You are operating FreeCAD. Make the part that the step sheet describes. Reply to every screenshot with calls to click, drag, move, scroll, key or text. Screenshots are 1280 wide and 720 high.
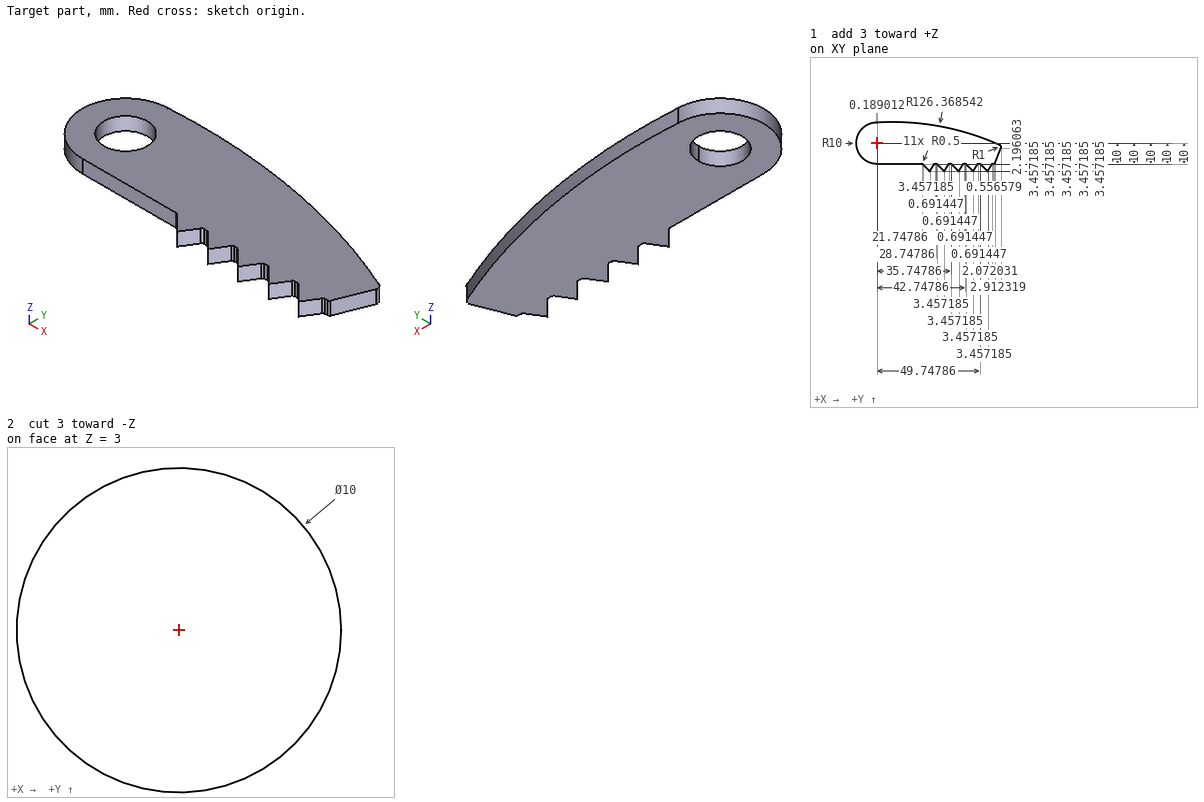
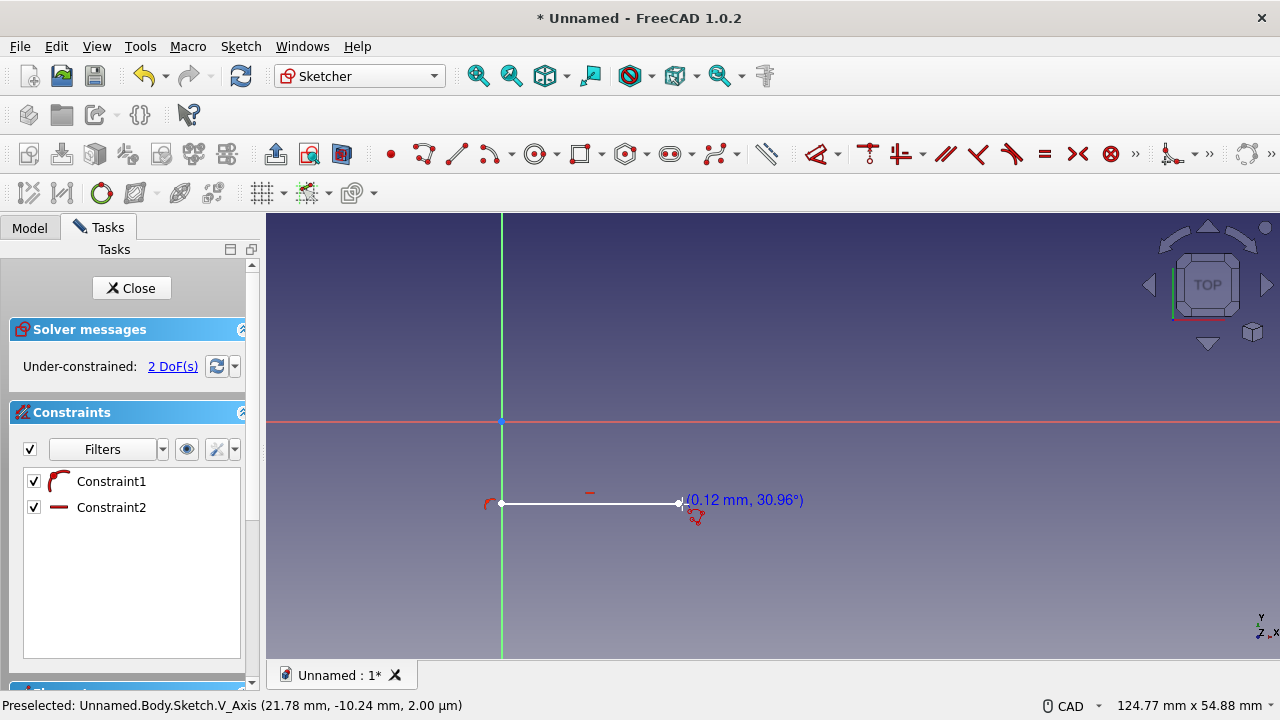
click(710, 532)
click(726, 505)
right_click(726, 505)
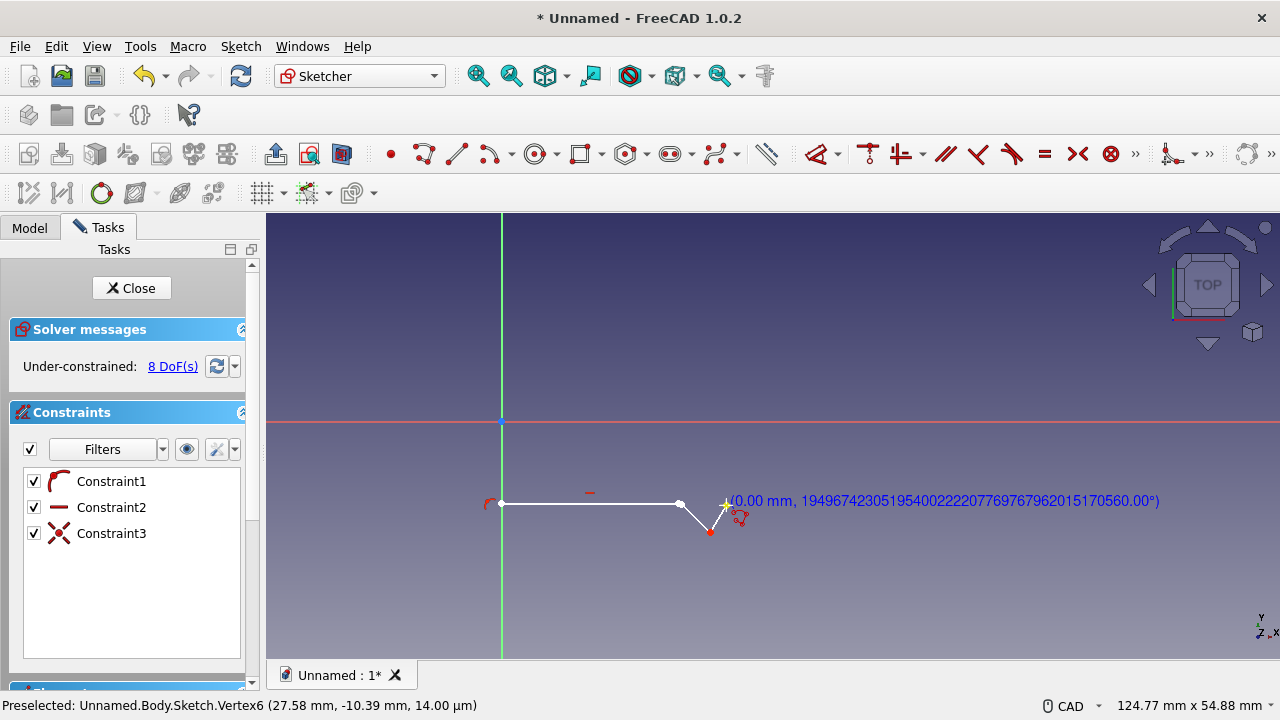
click(457, 154)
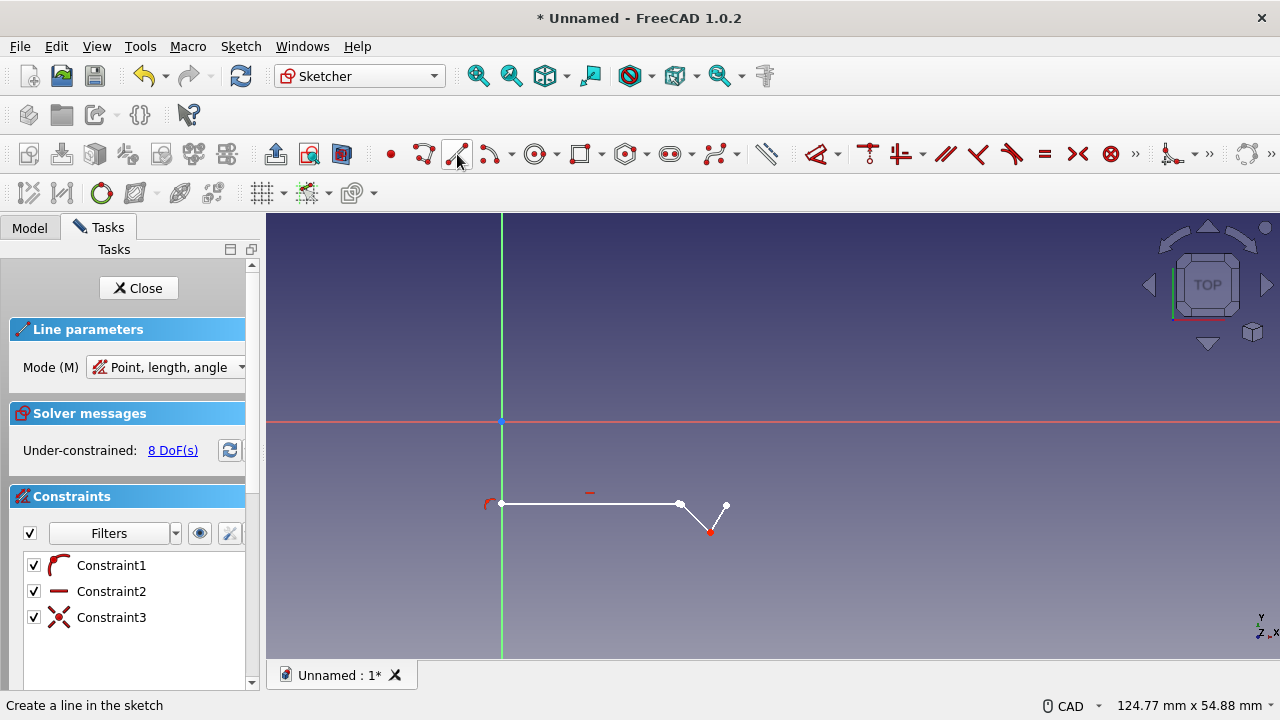
scroll(730, 503, up, 7)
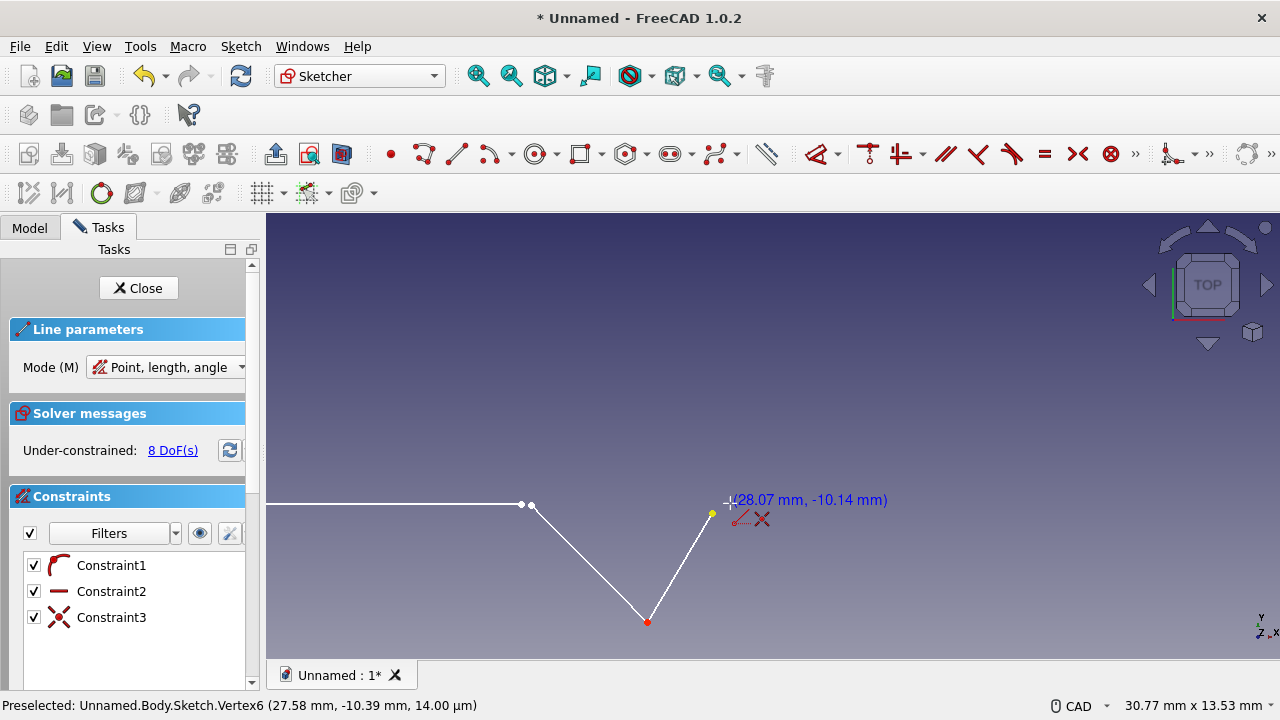
click(728, 500)
click(751, 500)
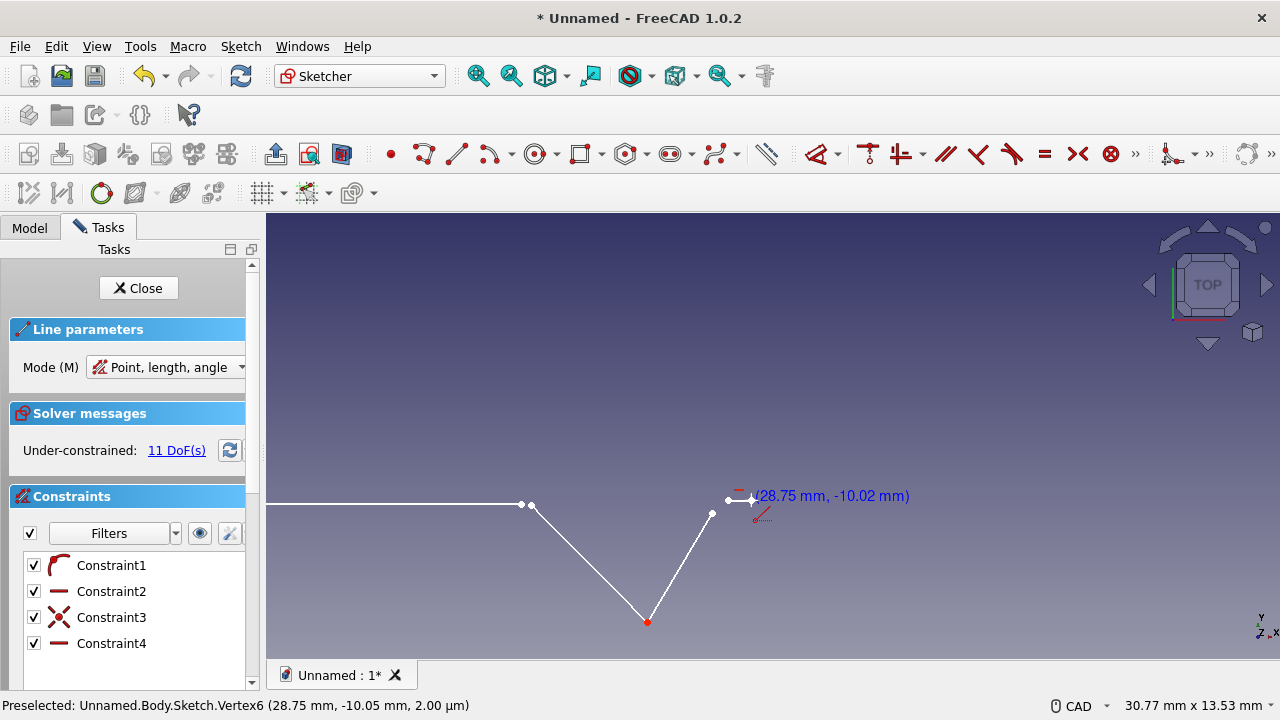
click(424, 154)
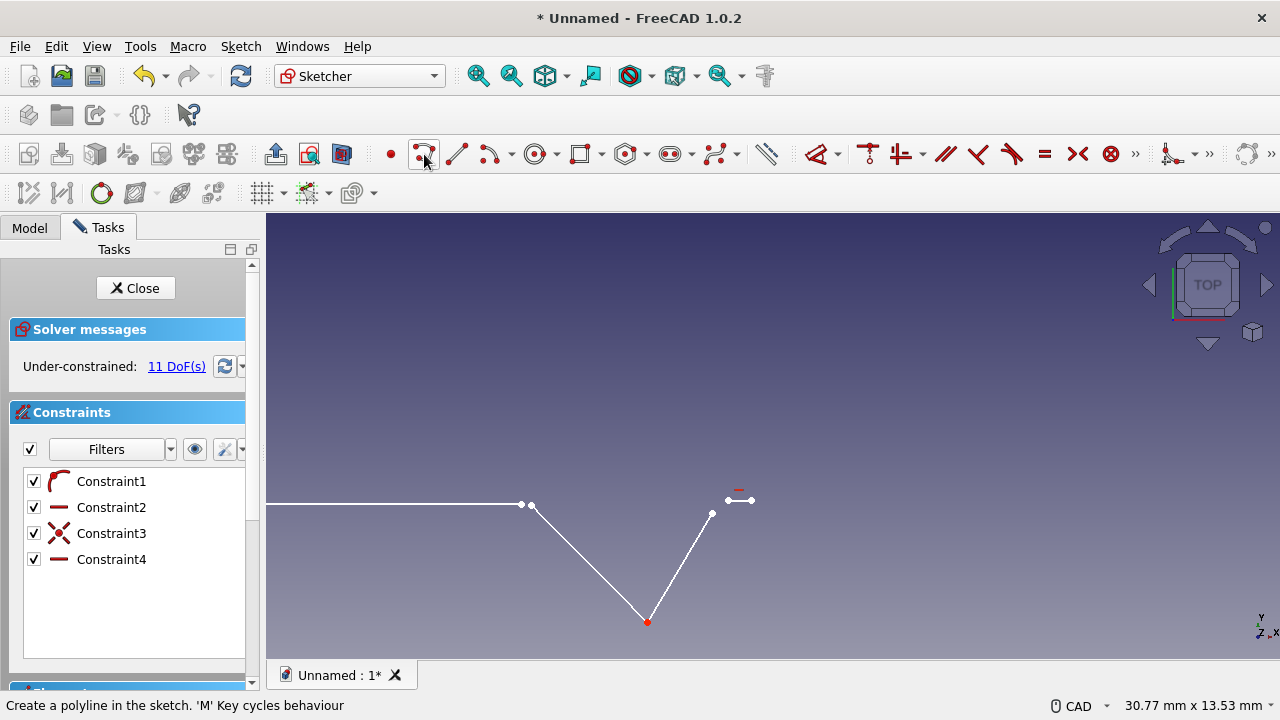
scroll(762, 505, up, 2)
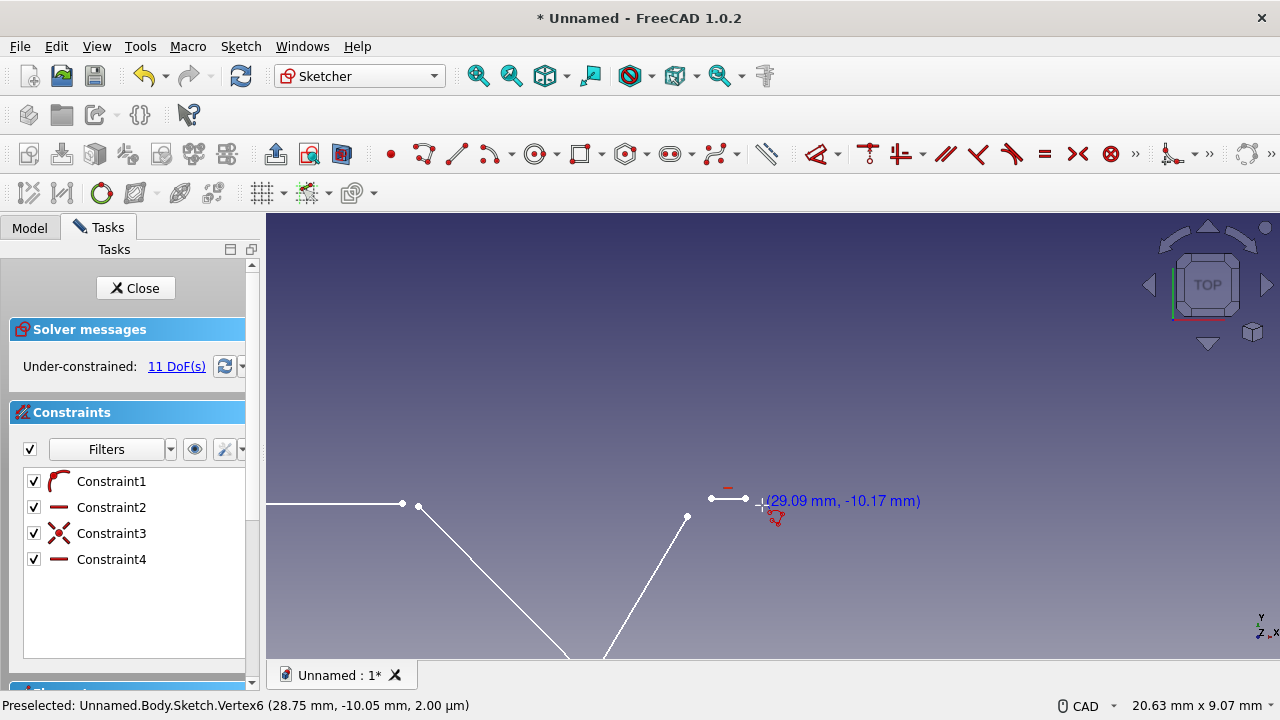
click(762, 505)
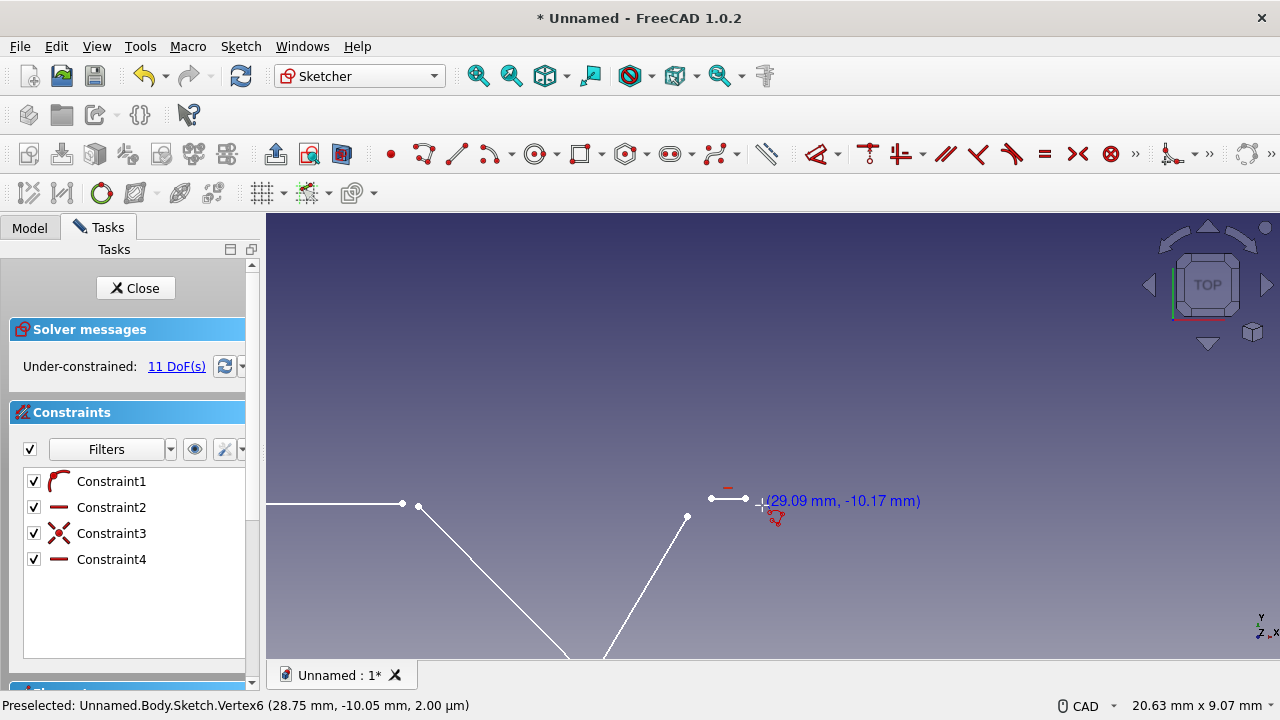
scroll(733, 504, down, 9)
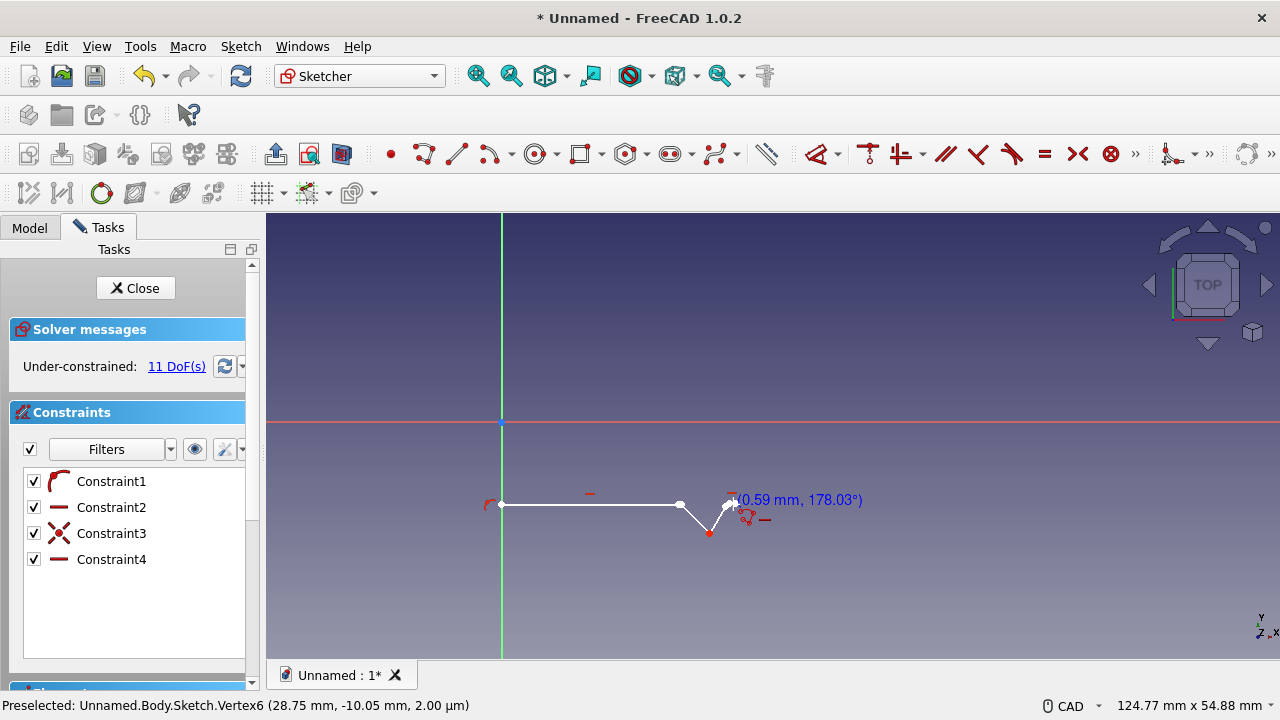
click(766, 533)
click(783, 505)
right_click(783, 505)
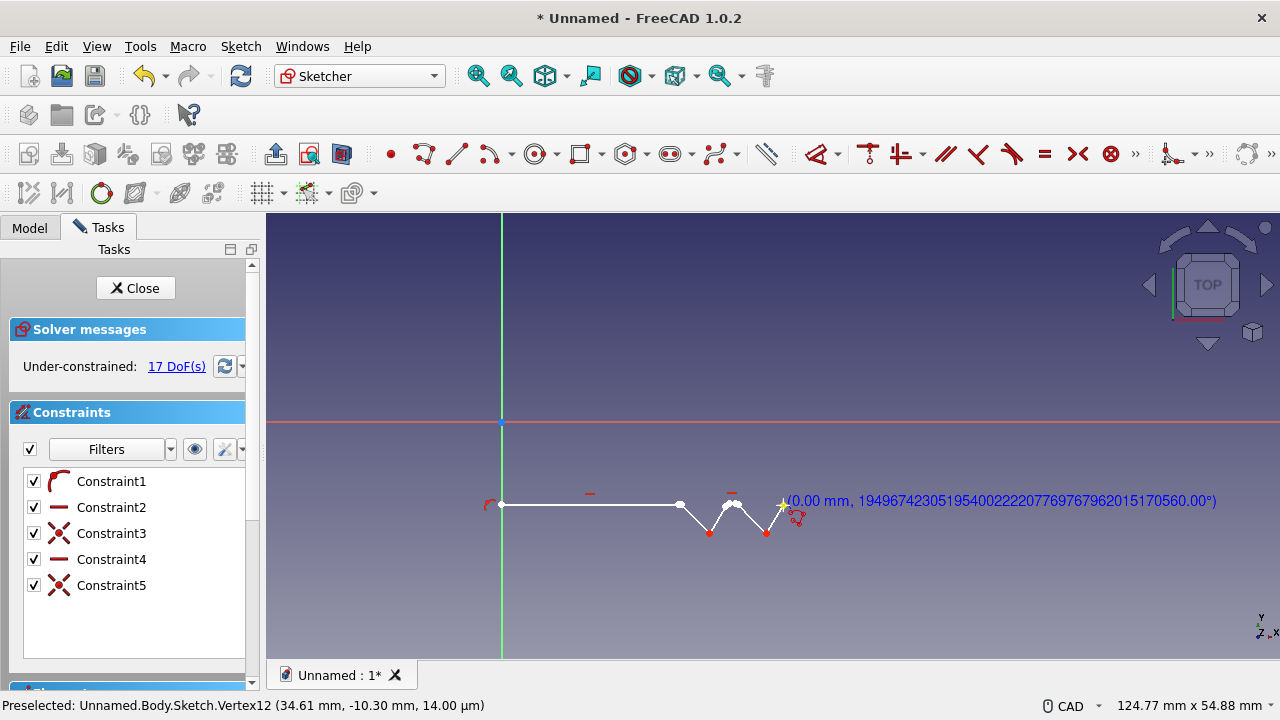
click(457, 154)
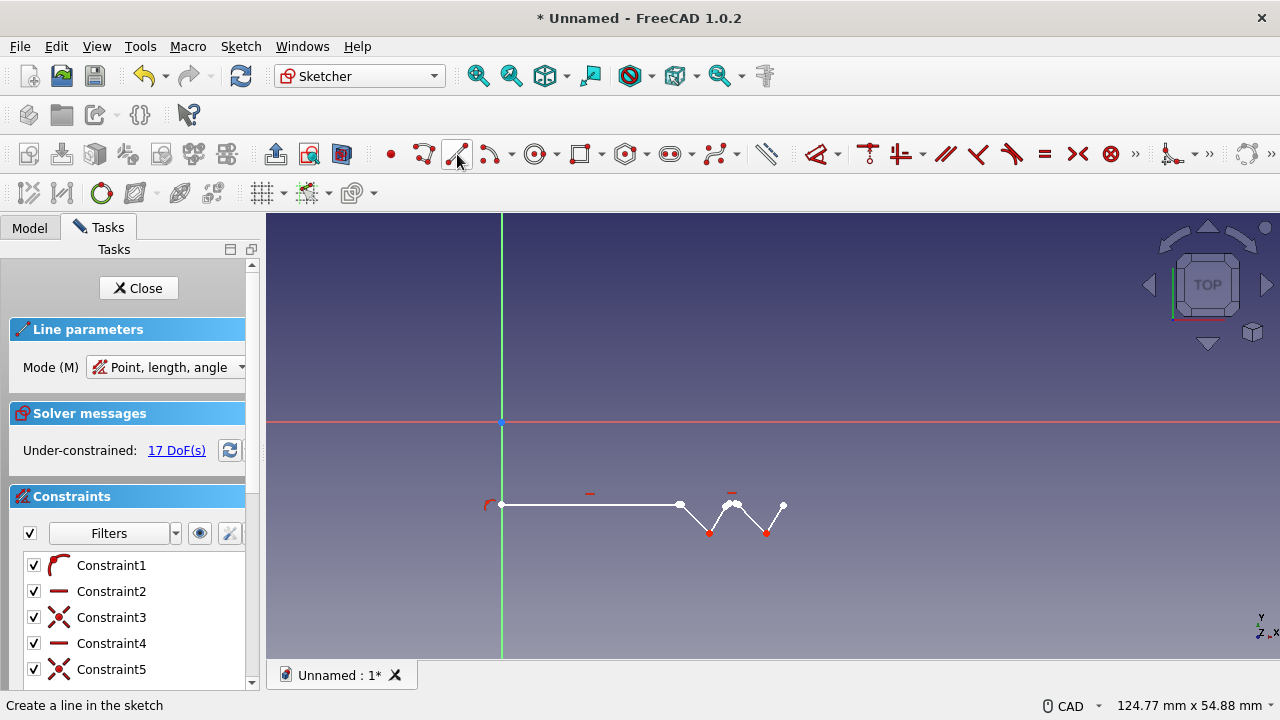
scroll(787, 504, up, 7)